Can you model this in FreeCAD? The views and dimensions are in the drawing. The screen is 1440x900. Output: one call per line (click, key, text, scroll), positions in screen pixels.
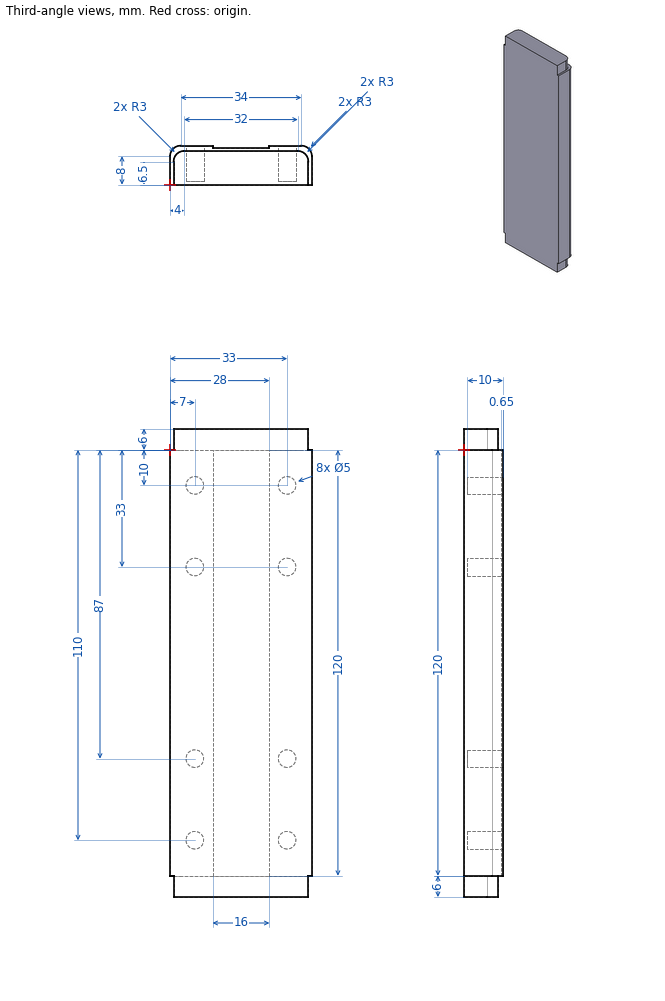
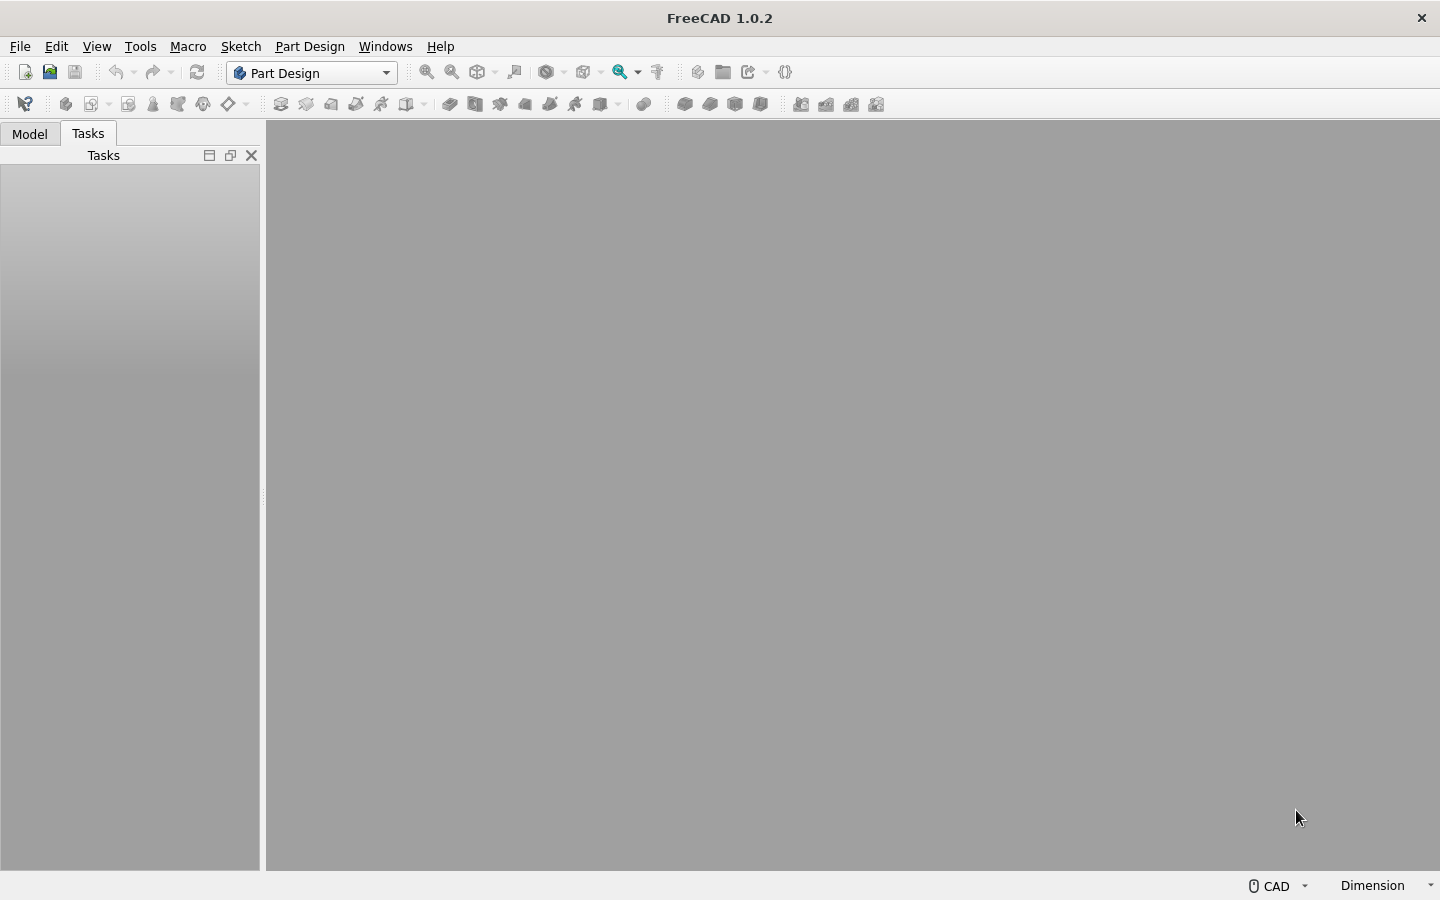
click(25, 72)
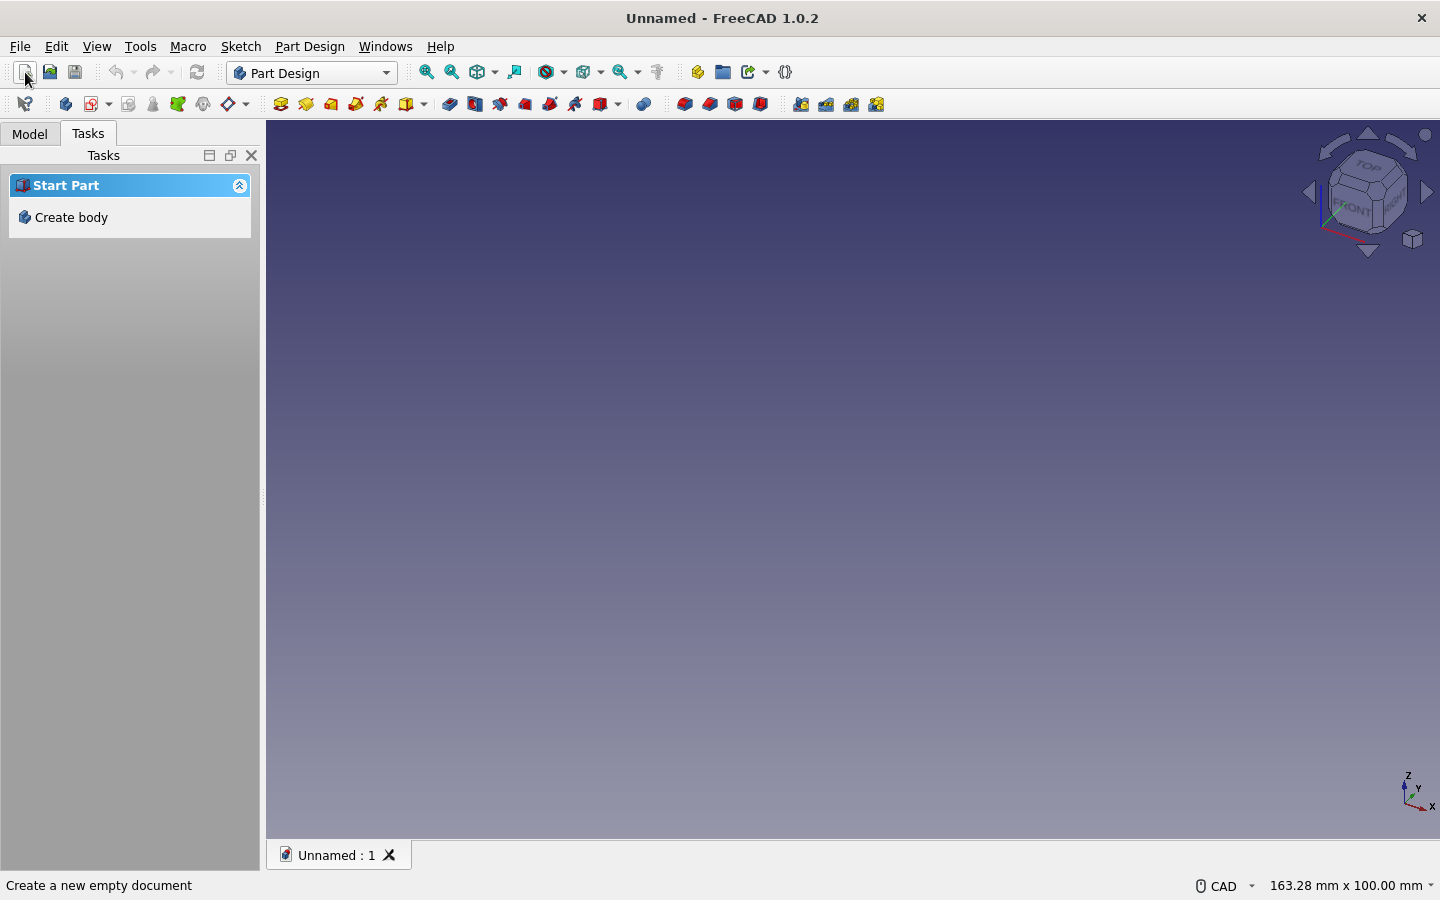
click(90, 104)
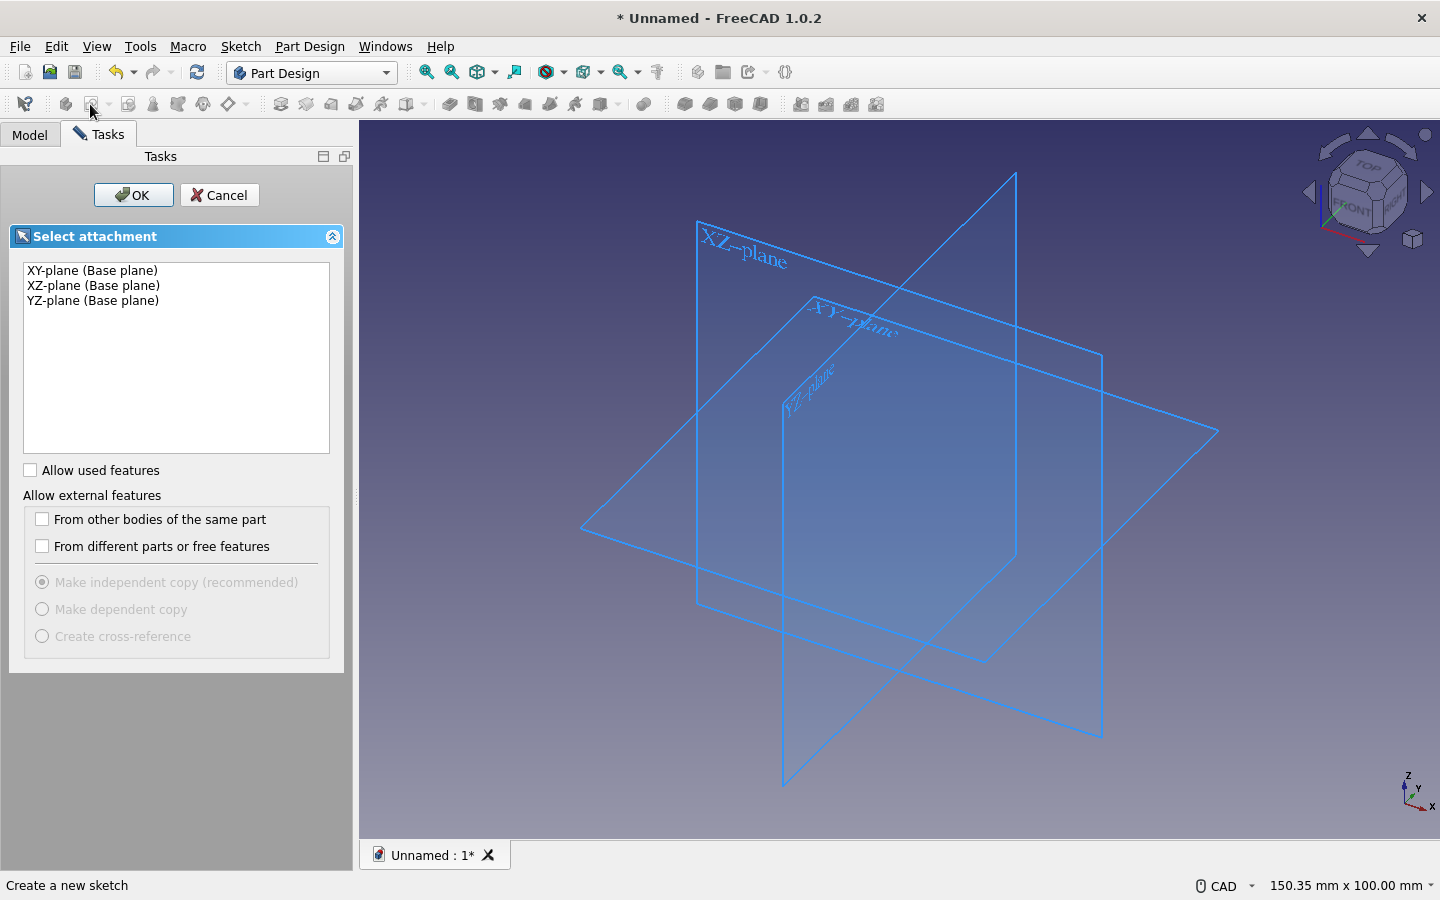
click(84, 270)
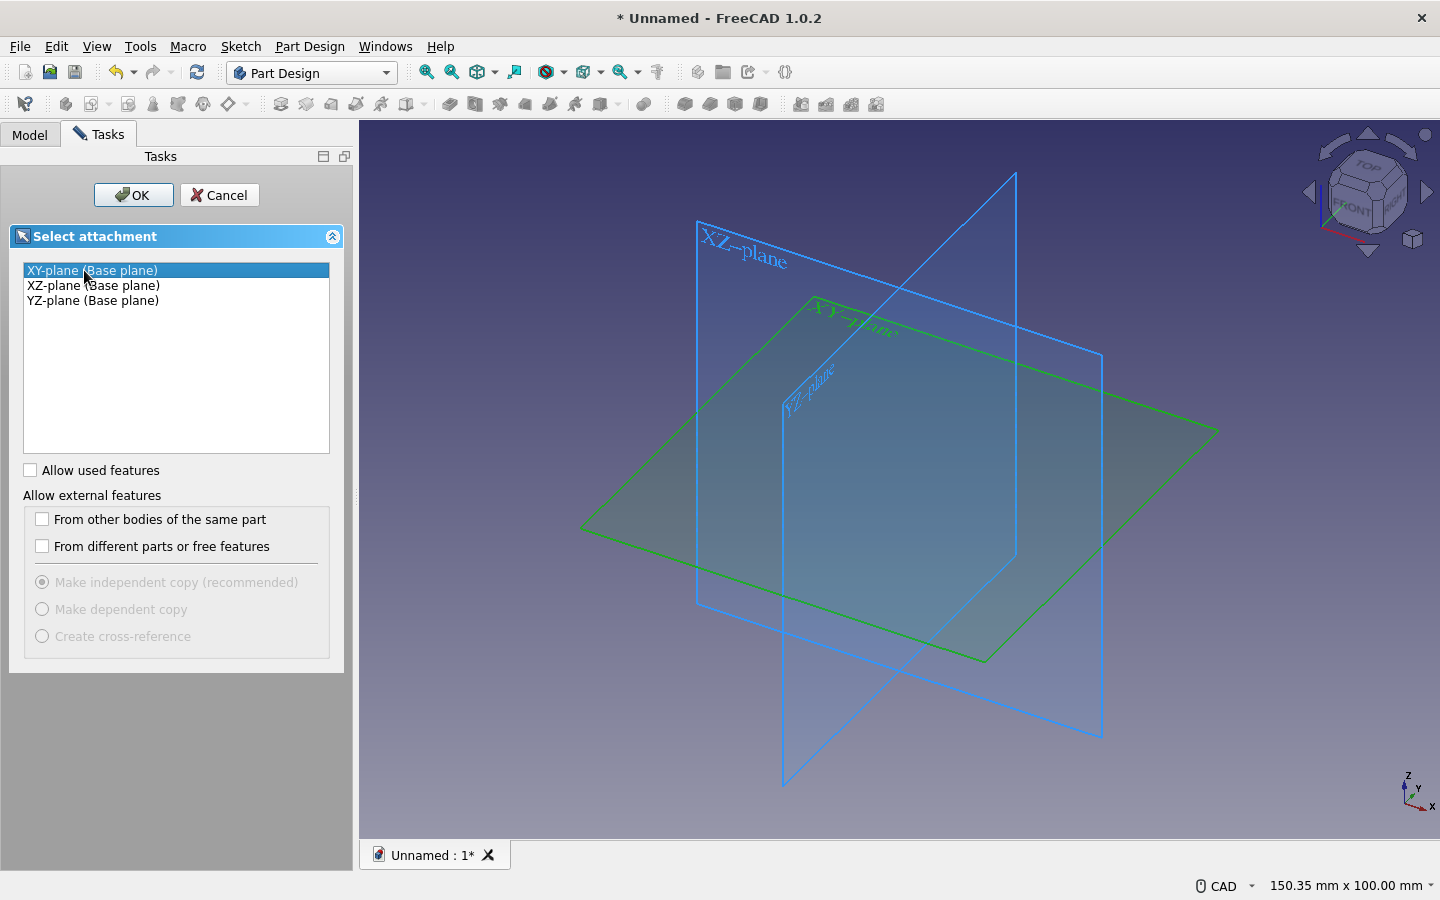
click(134, 195)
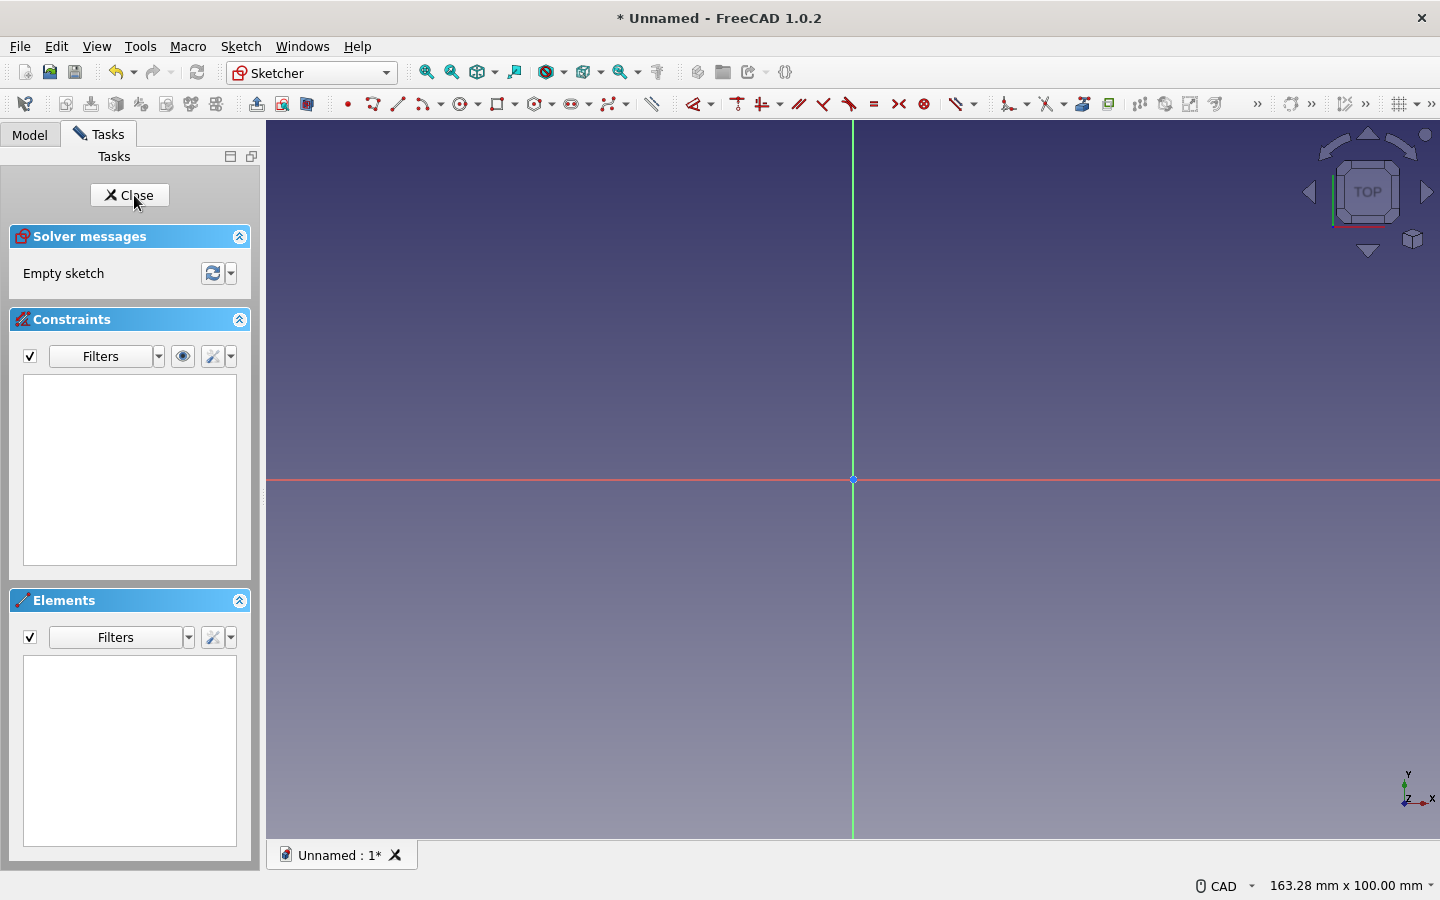
scroll(1170, 408, up, 4)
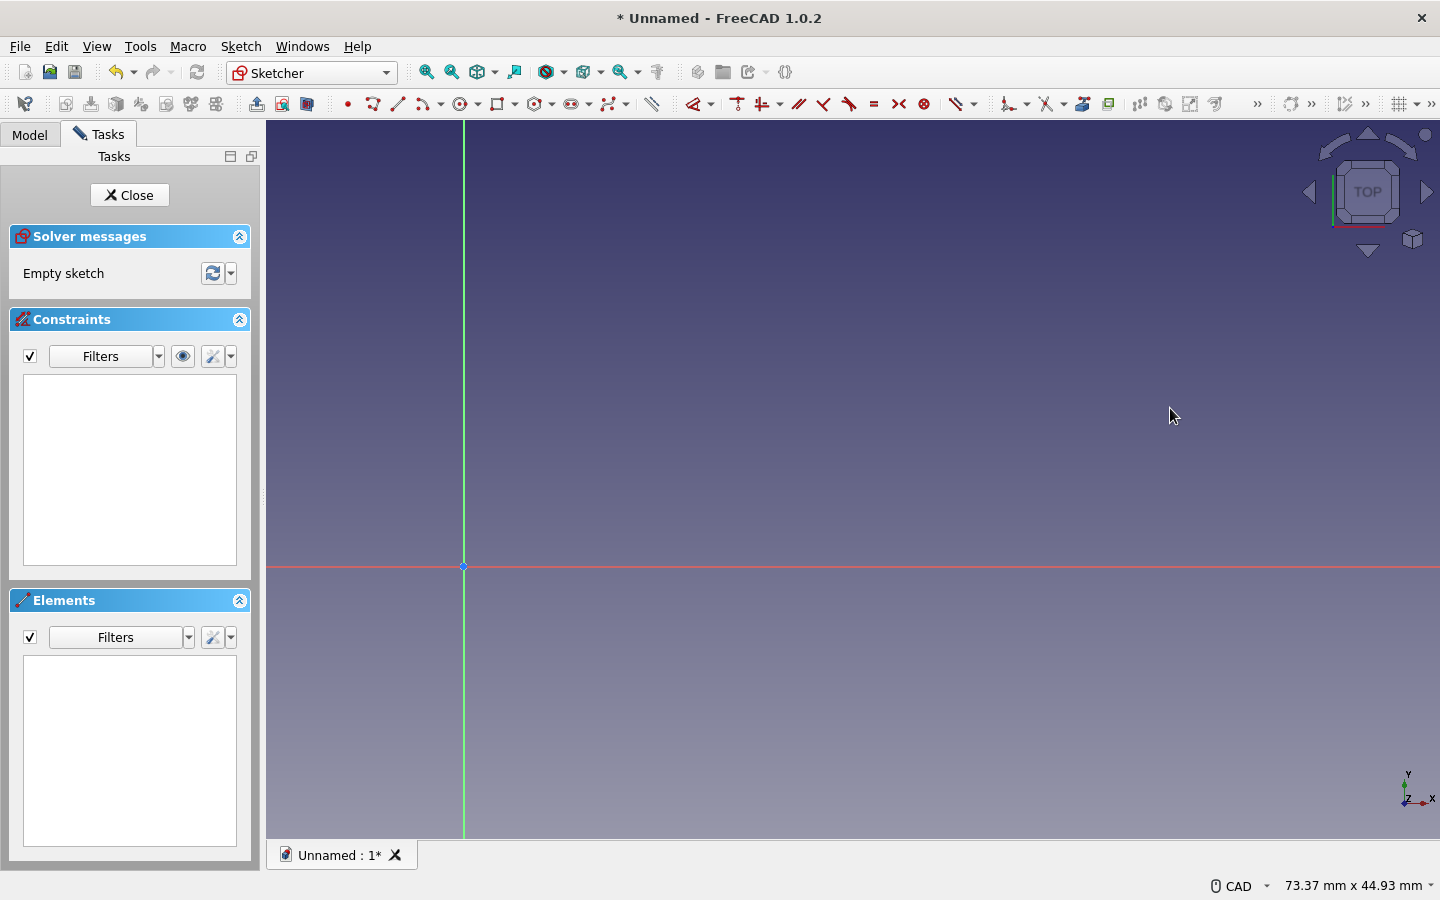
click(398, 104)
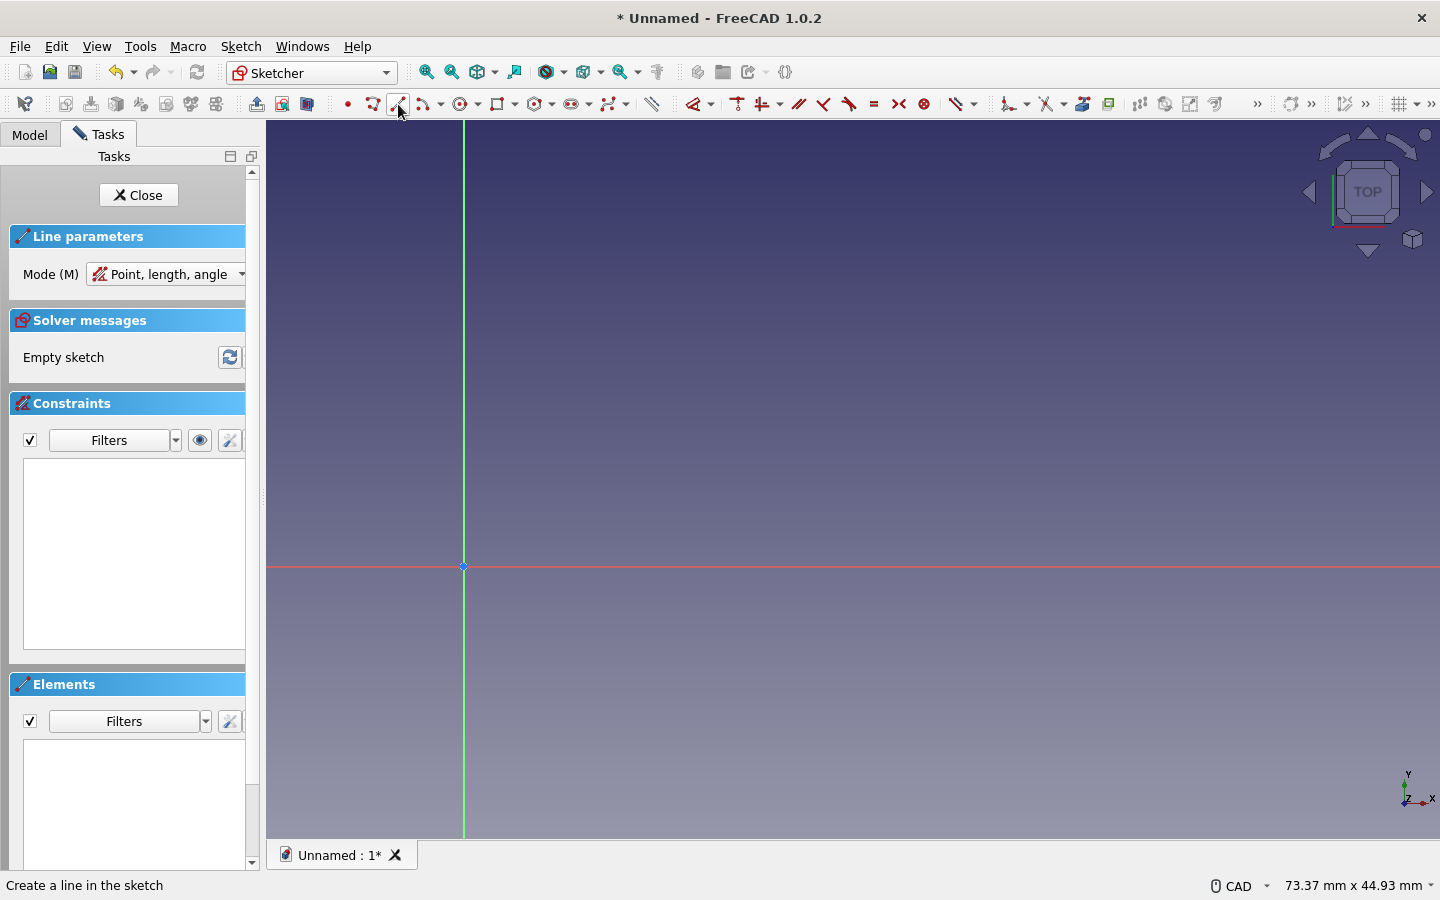
click(1056, 391)
click(512, 391)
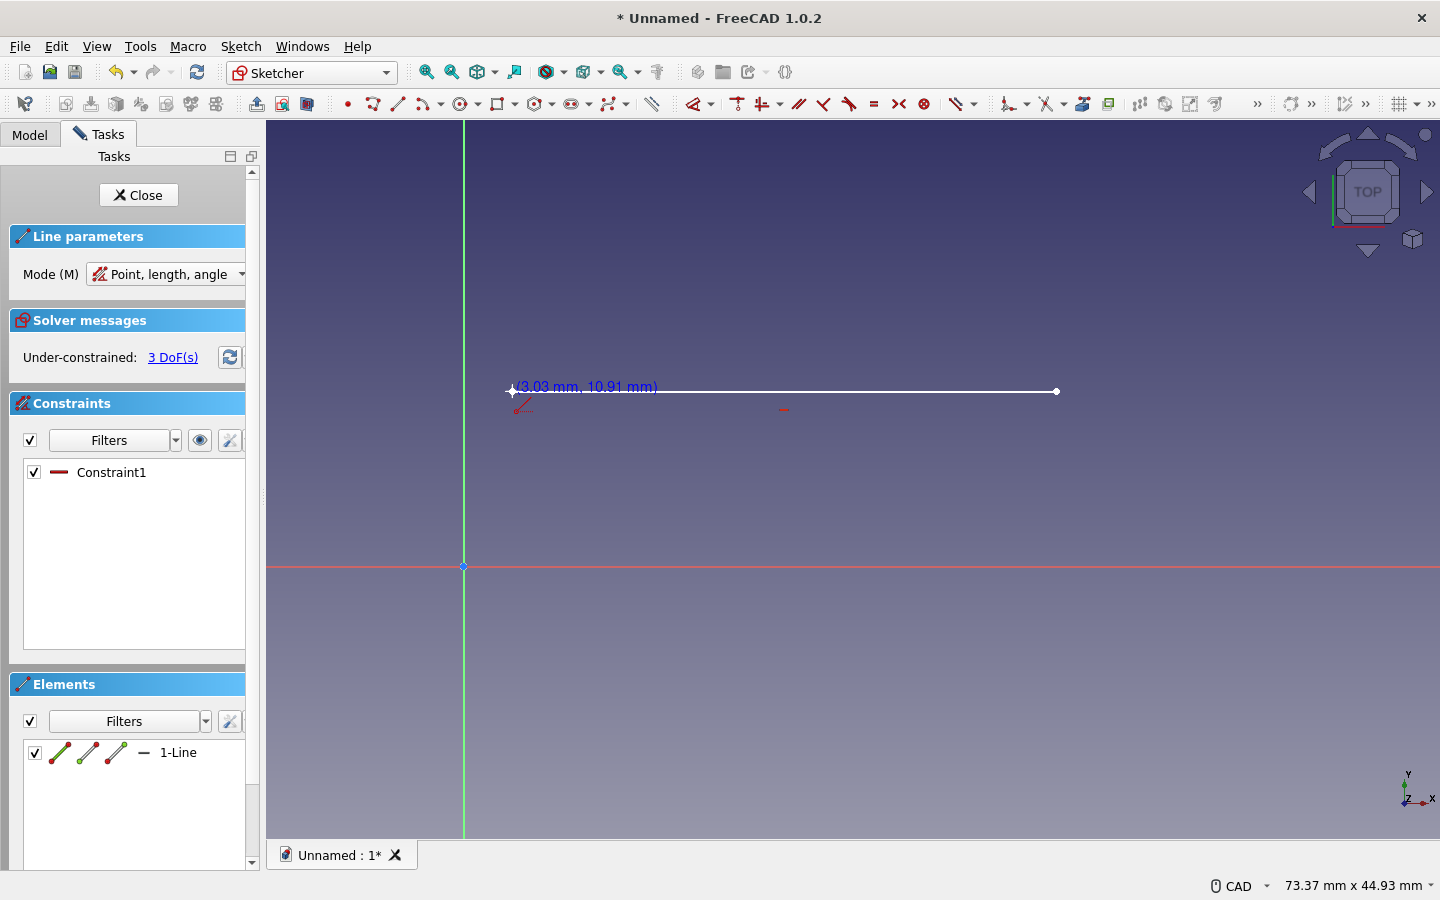
click(373, 104)